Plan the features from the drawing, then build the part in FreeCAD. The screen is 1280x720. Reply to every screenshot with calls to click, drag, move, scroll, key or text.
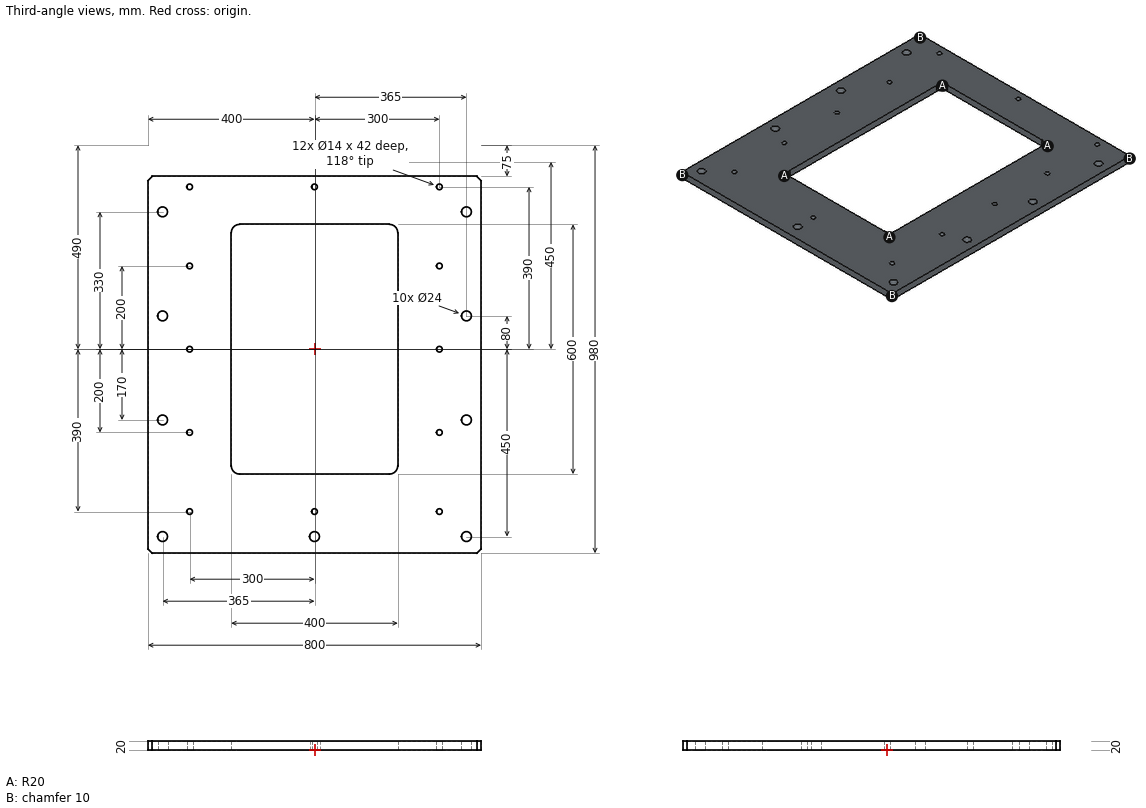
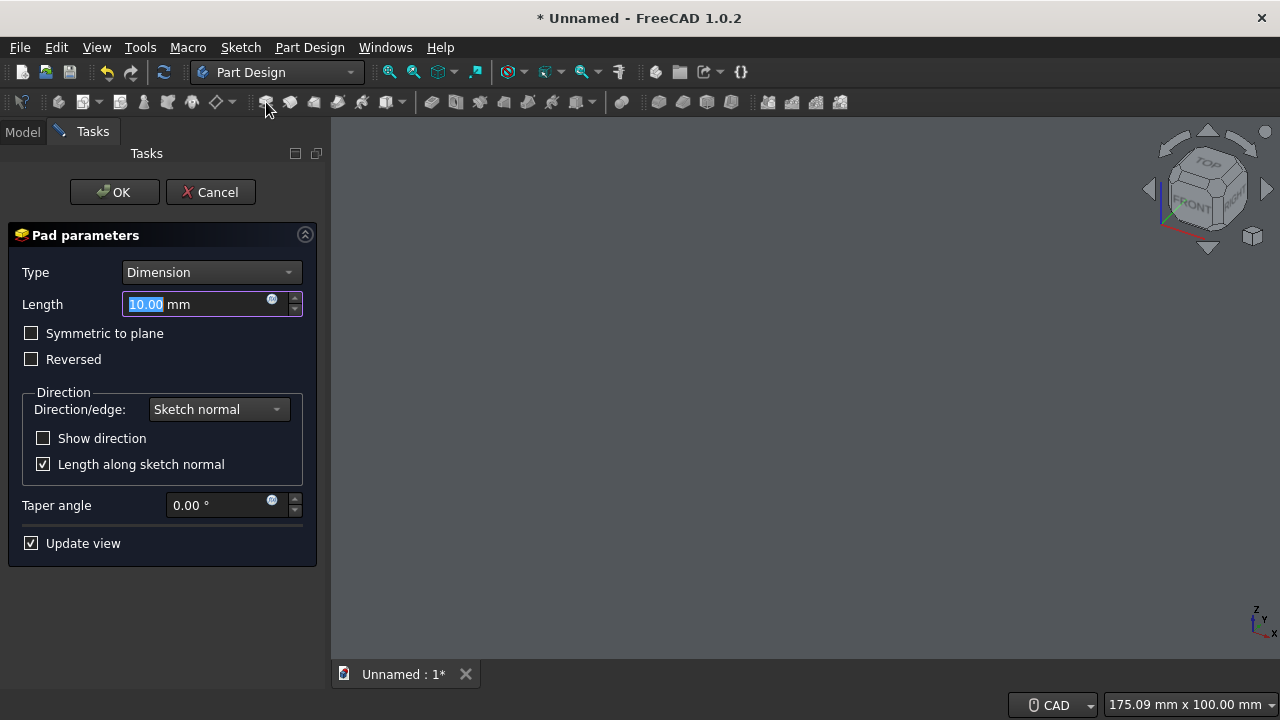
text(20)
key(Tab)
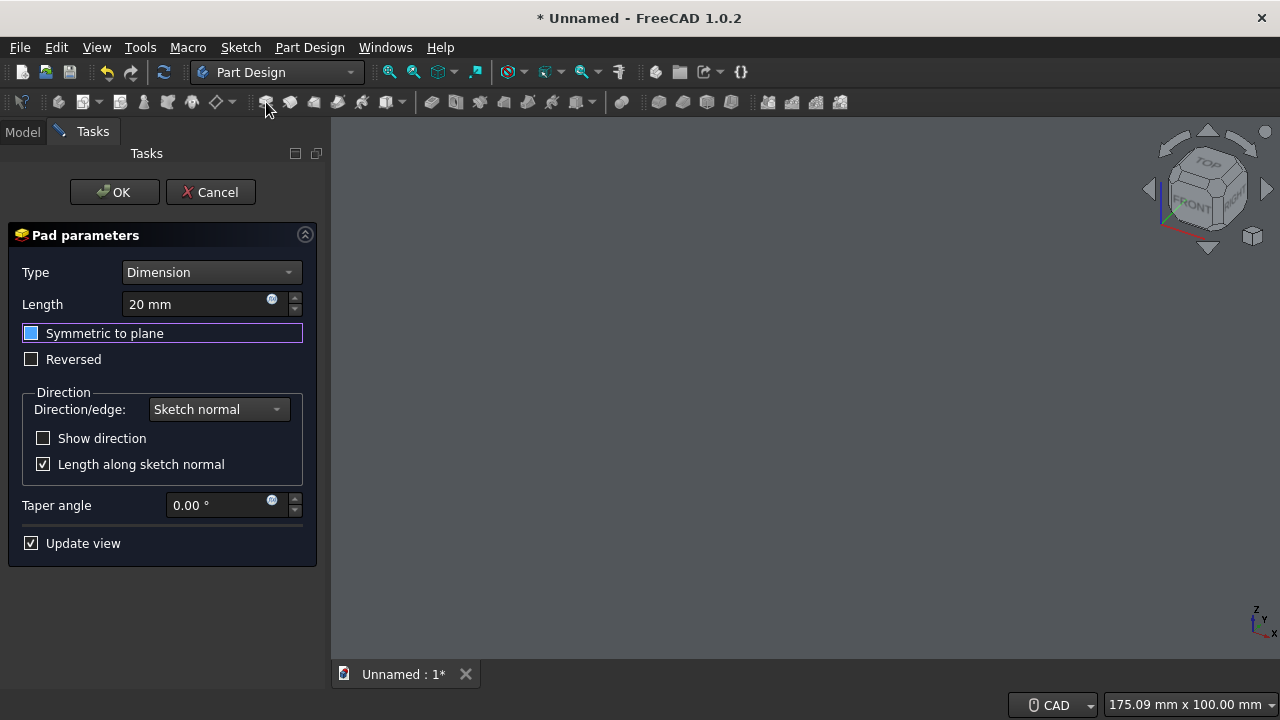
click(115, 192)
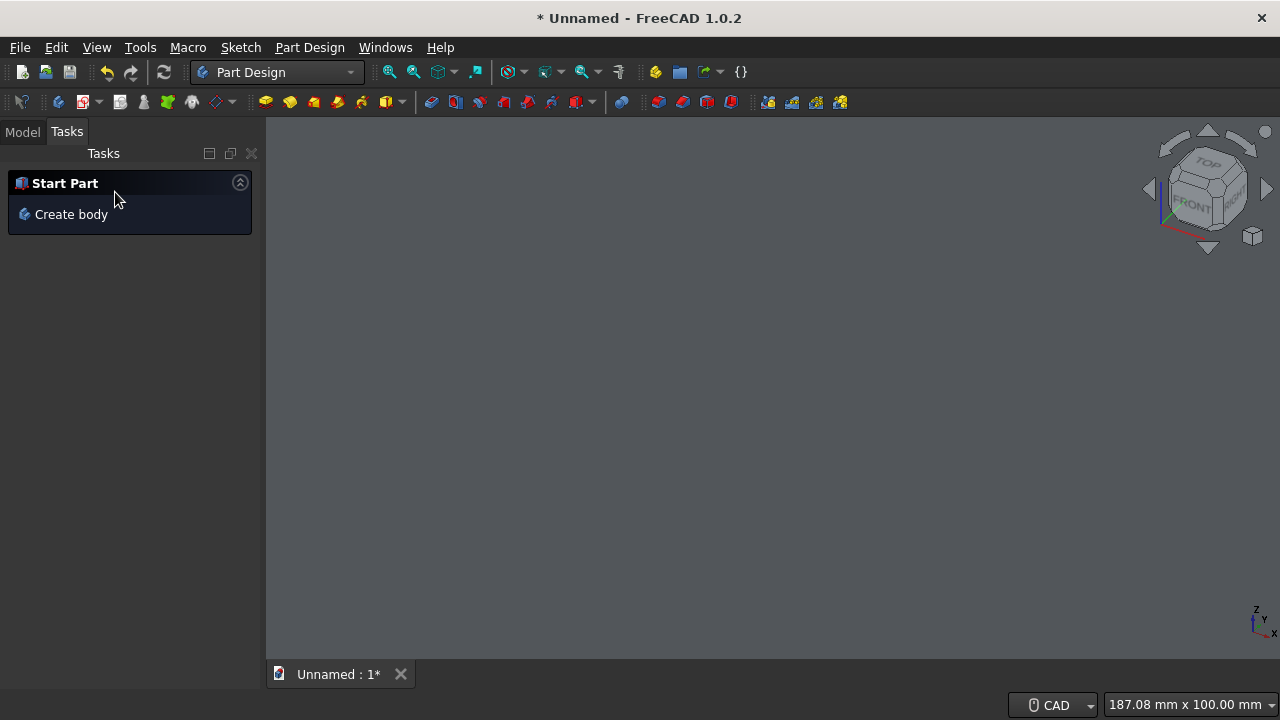
click(390, 72)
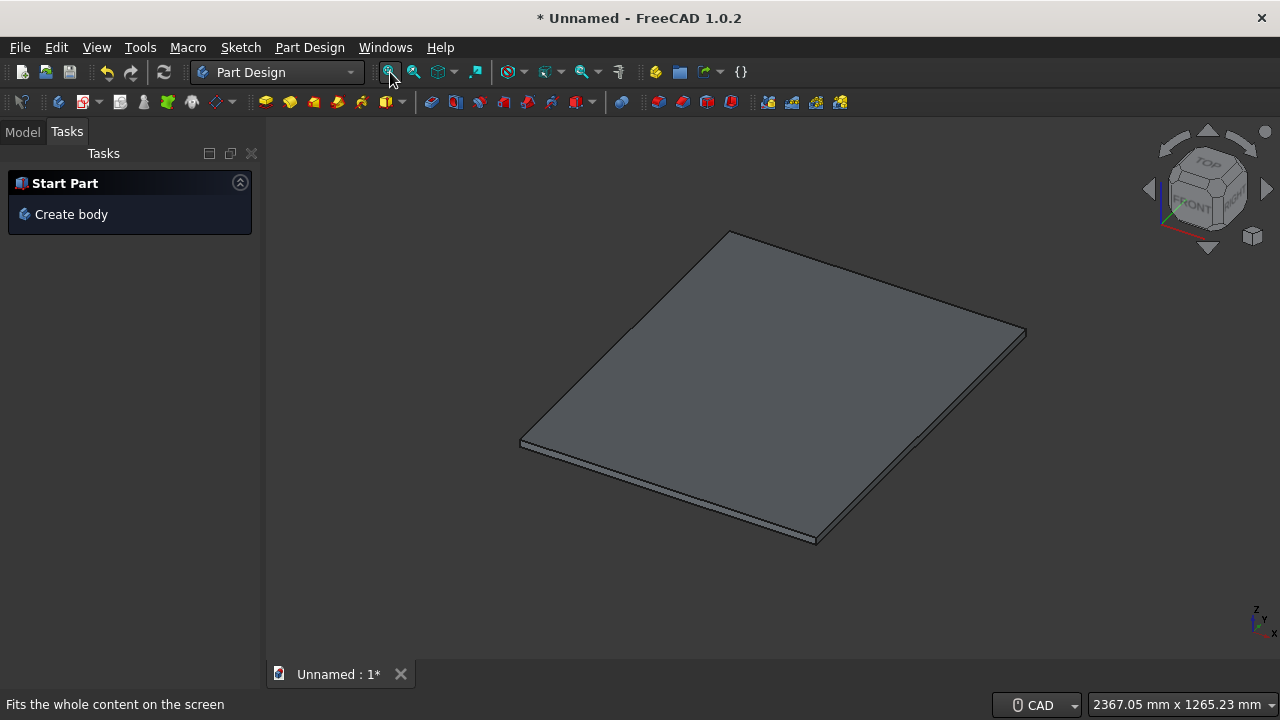
click(773, 383)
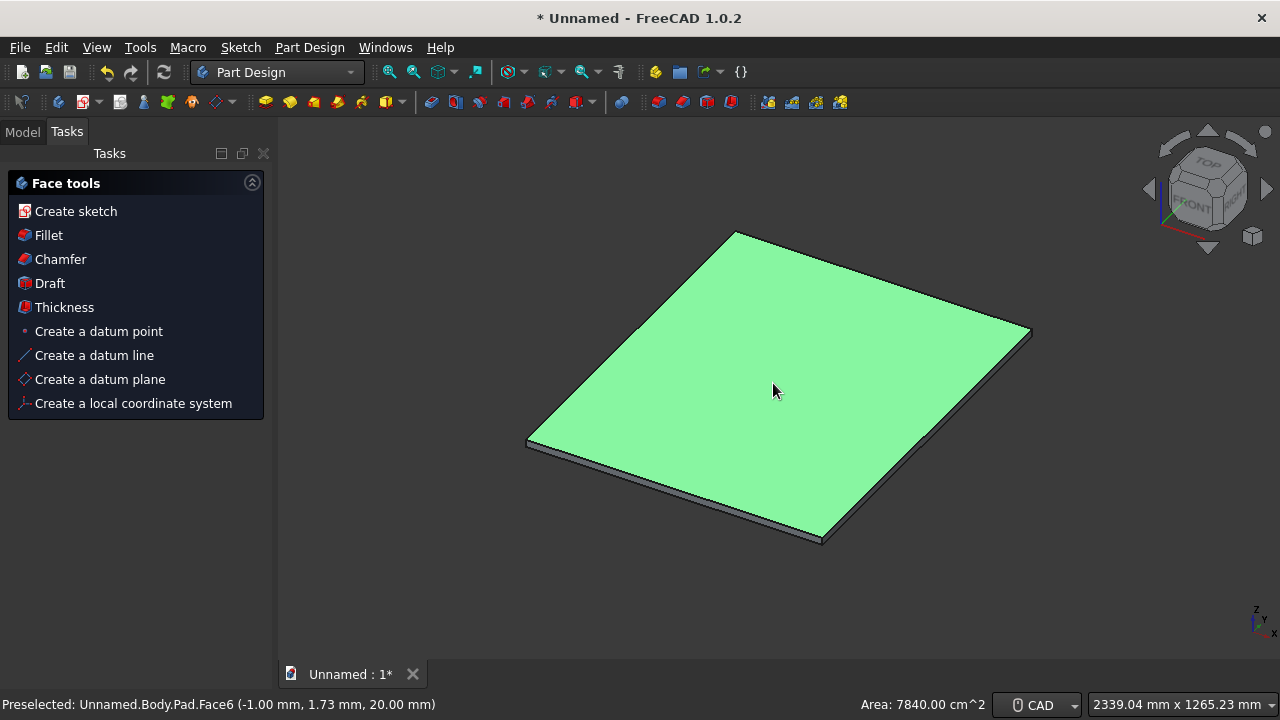
click(84, 102)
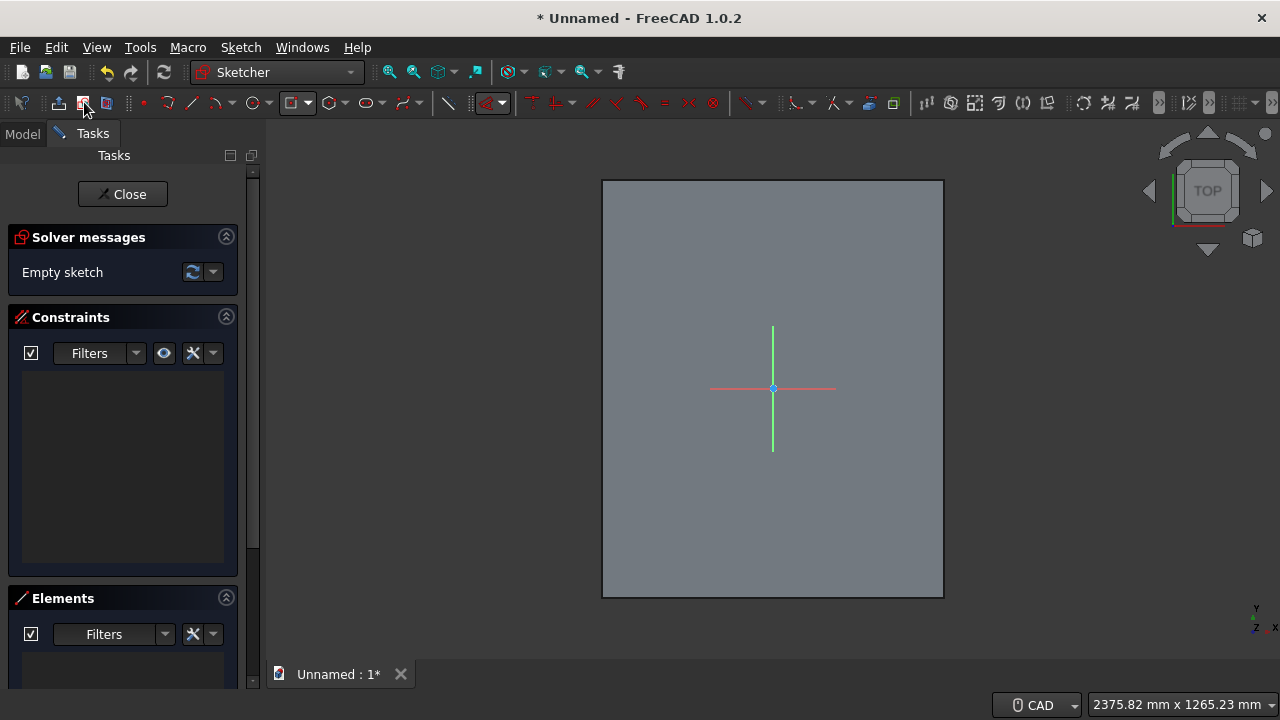
click(254, 104)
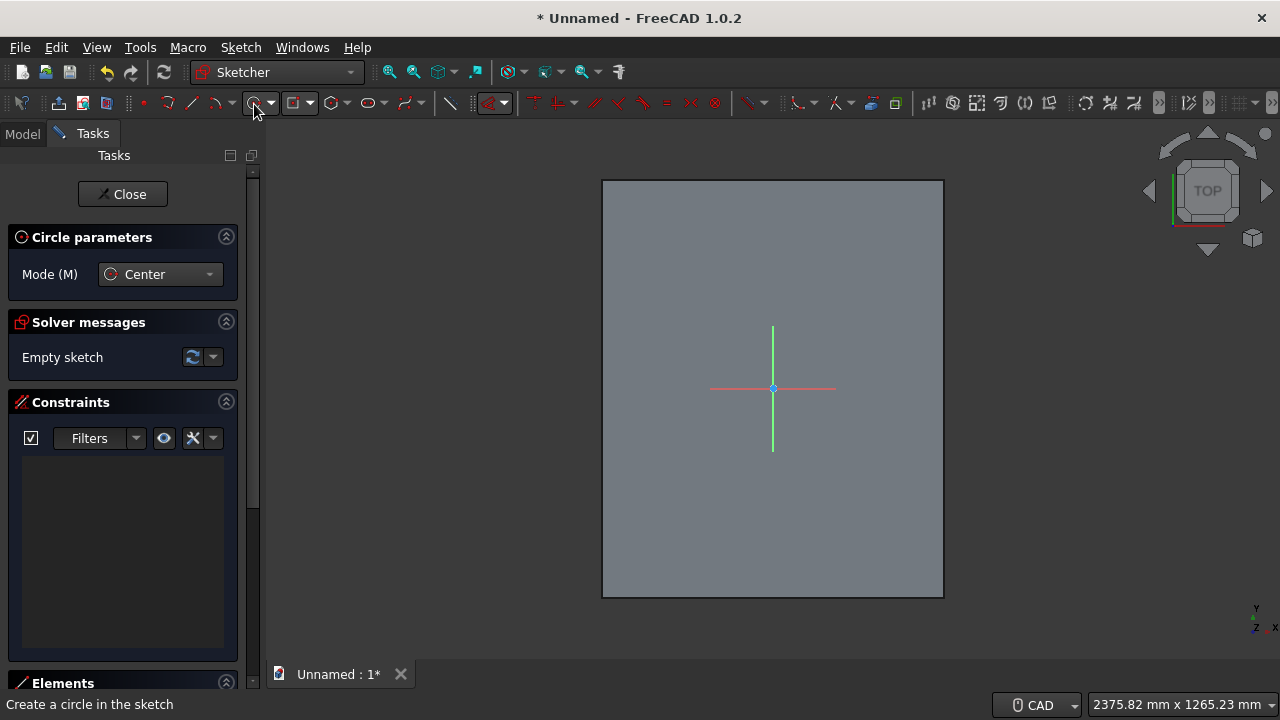
scroll(901, 223, up, 11)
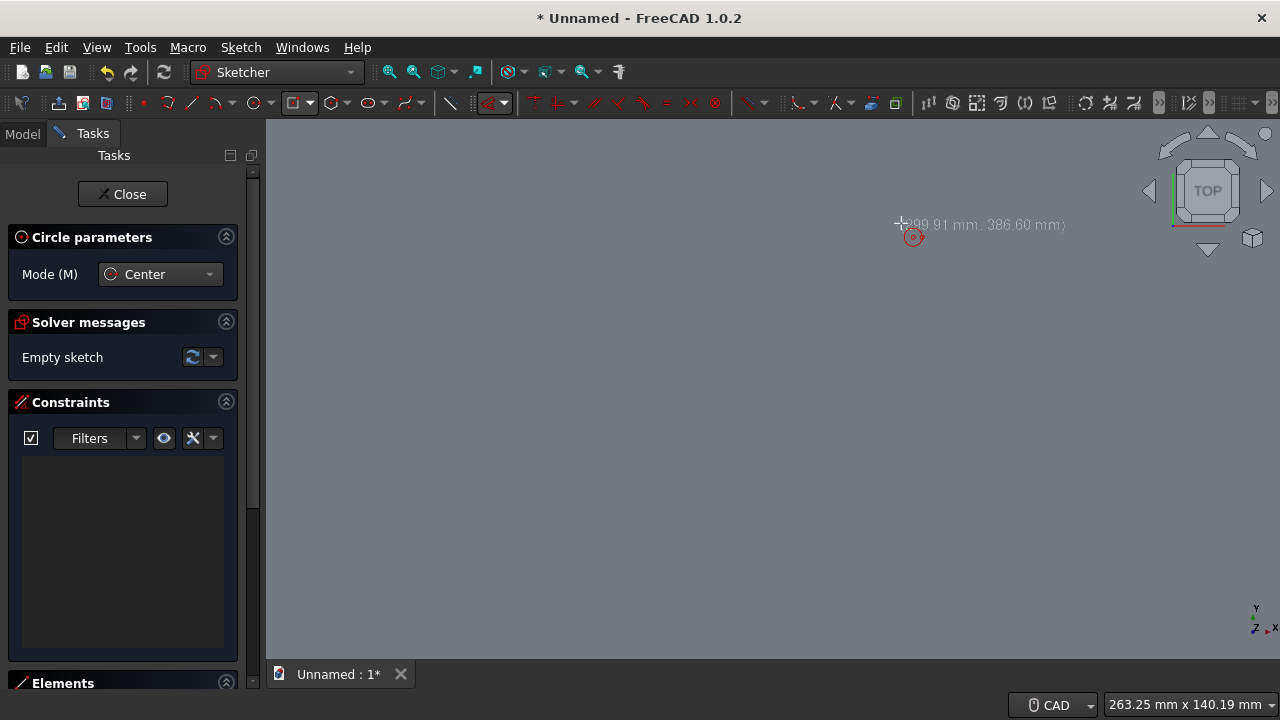
scroll(825, 223, down, 11)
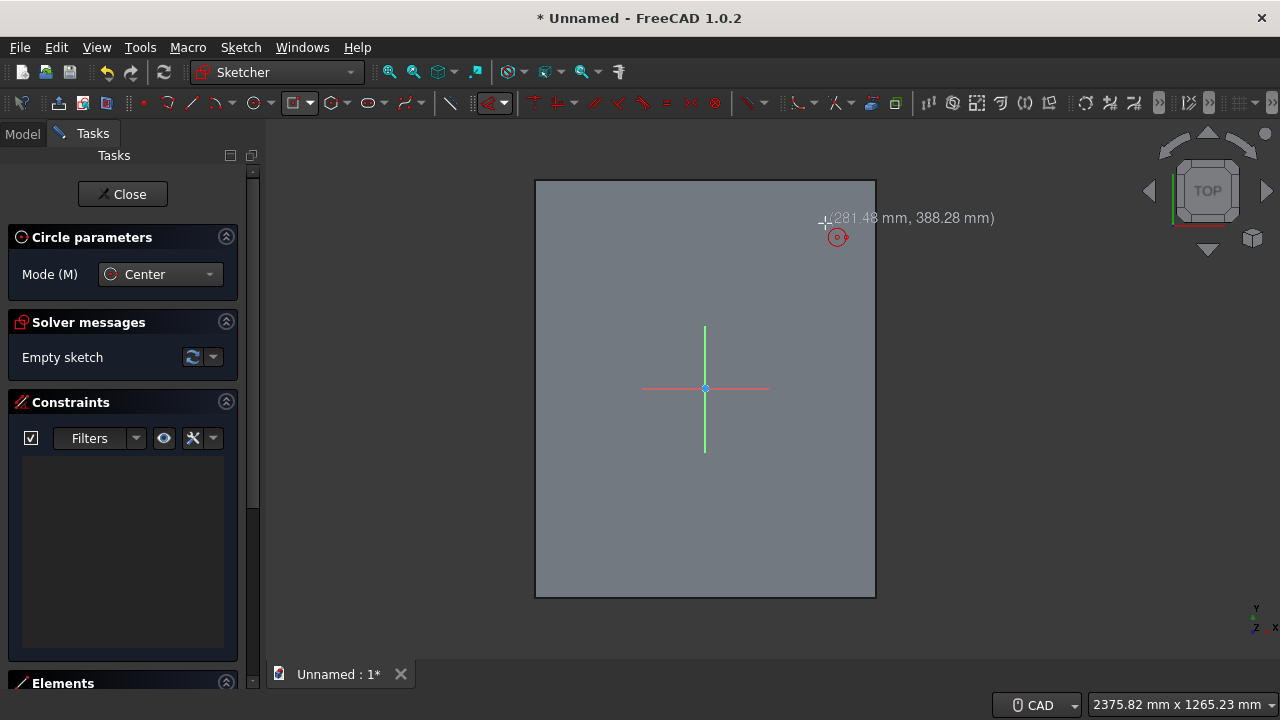
click(833, 223)
move(836, 220)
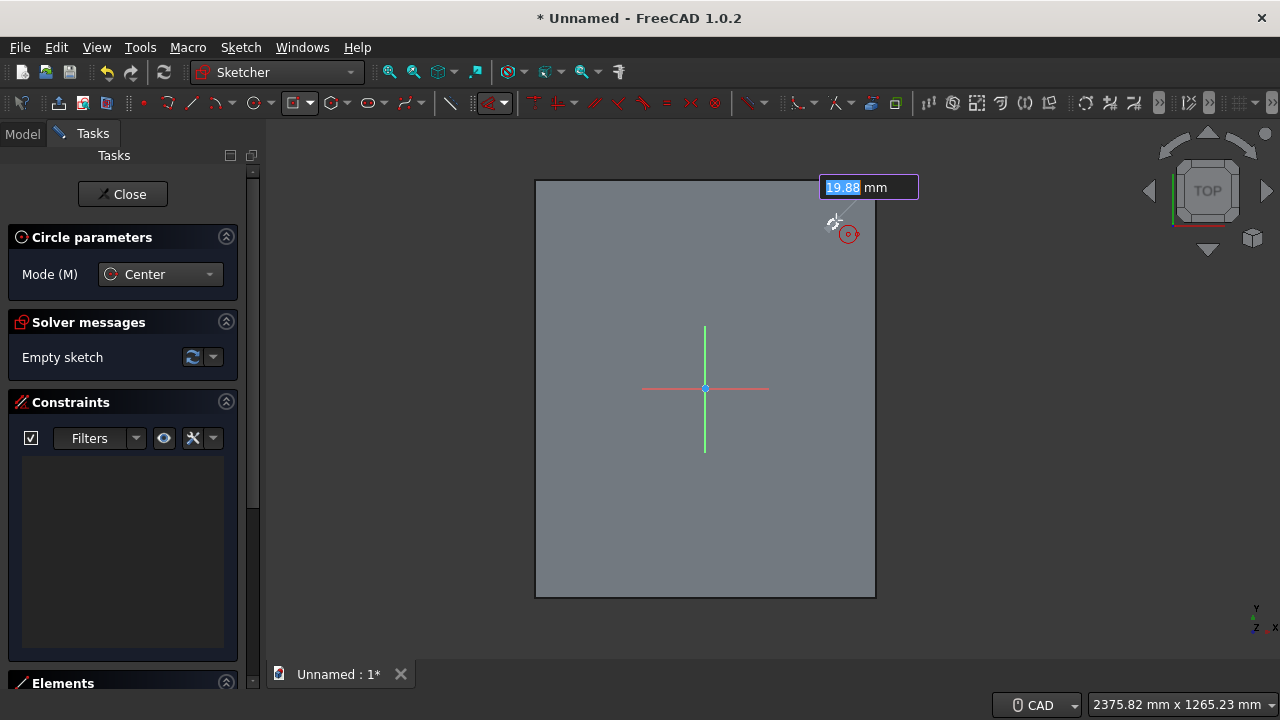
text(14)
key(Return)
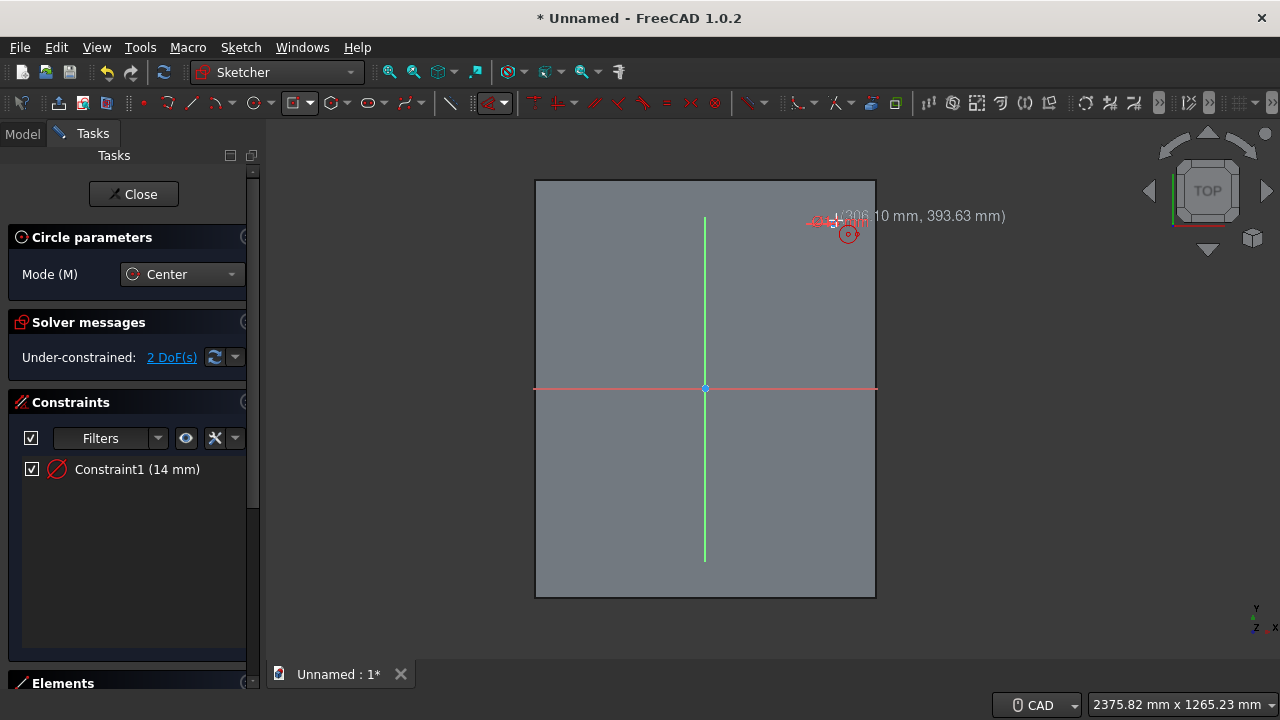
scroll(577, 555, up, 11)